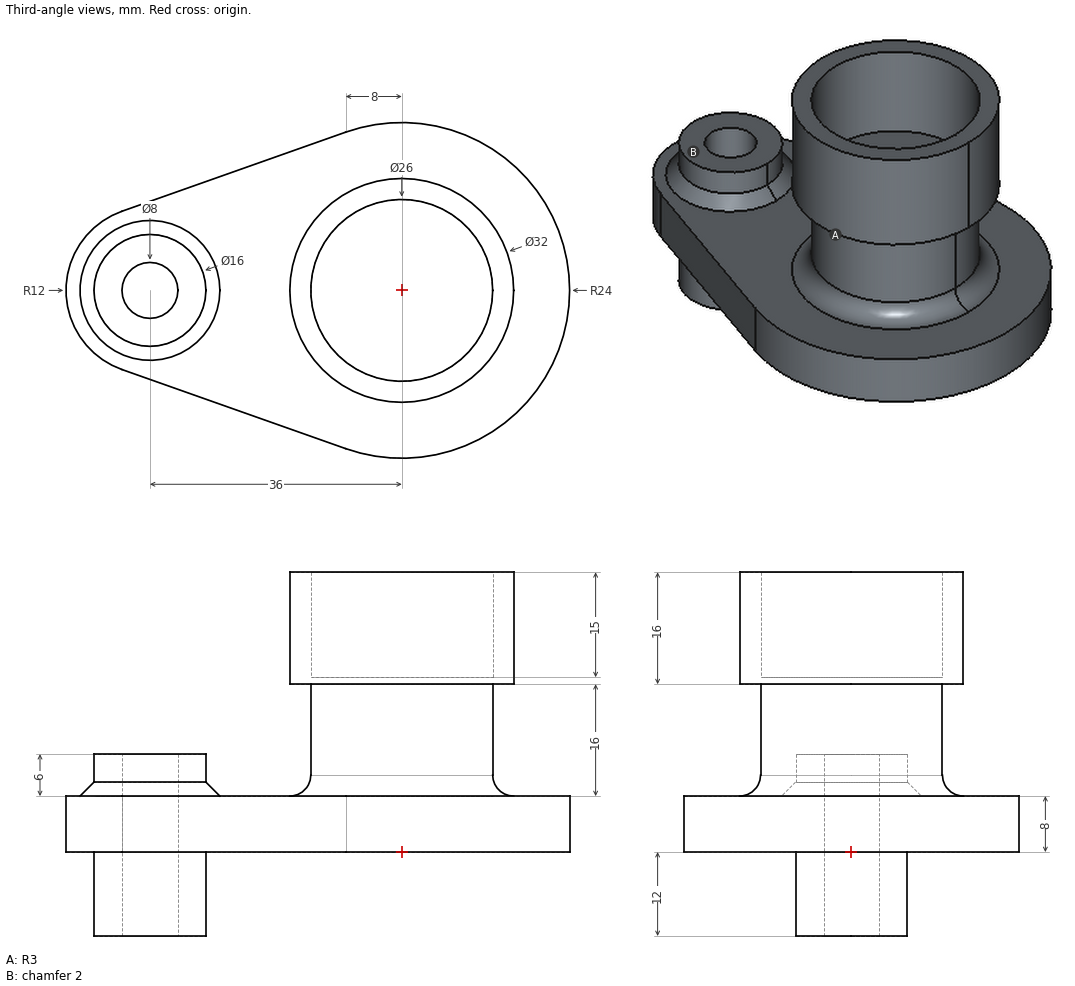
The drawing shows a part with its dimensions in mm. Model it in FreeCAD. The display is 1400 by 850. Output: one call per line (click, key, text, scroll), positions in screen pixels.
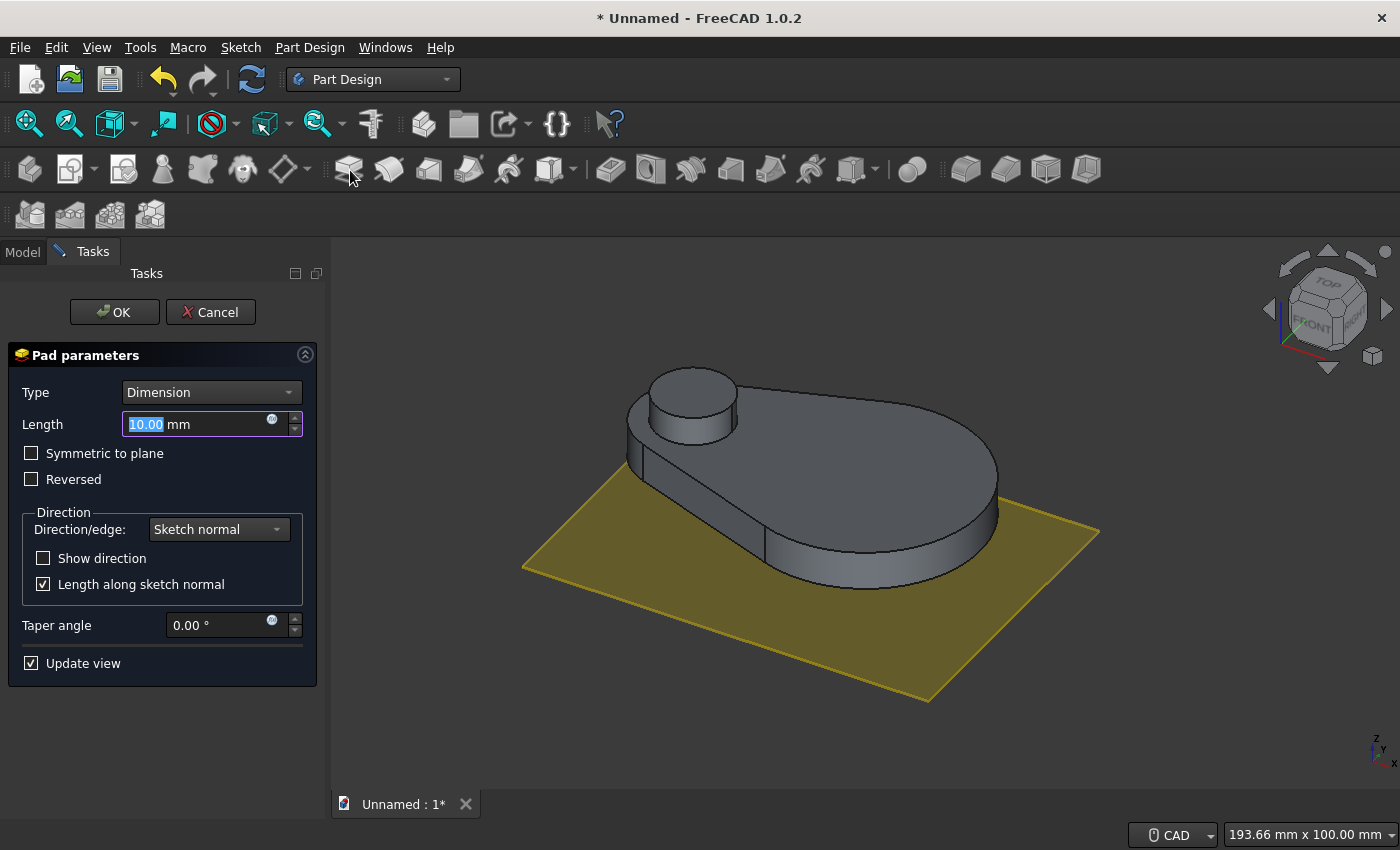
text(12)
key(Tab)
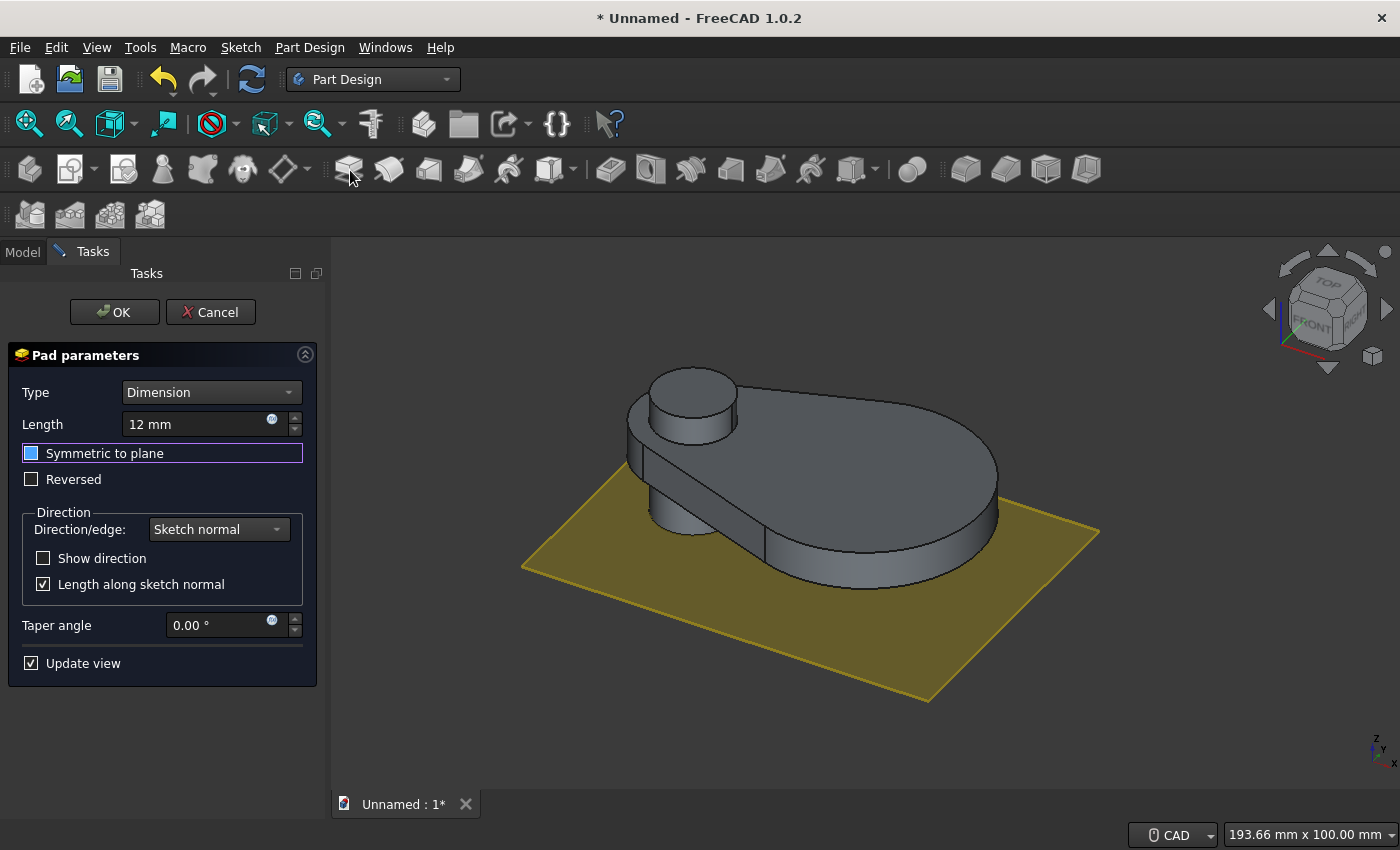
click(115, 312)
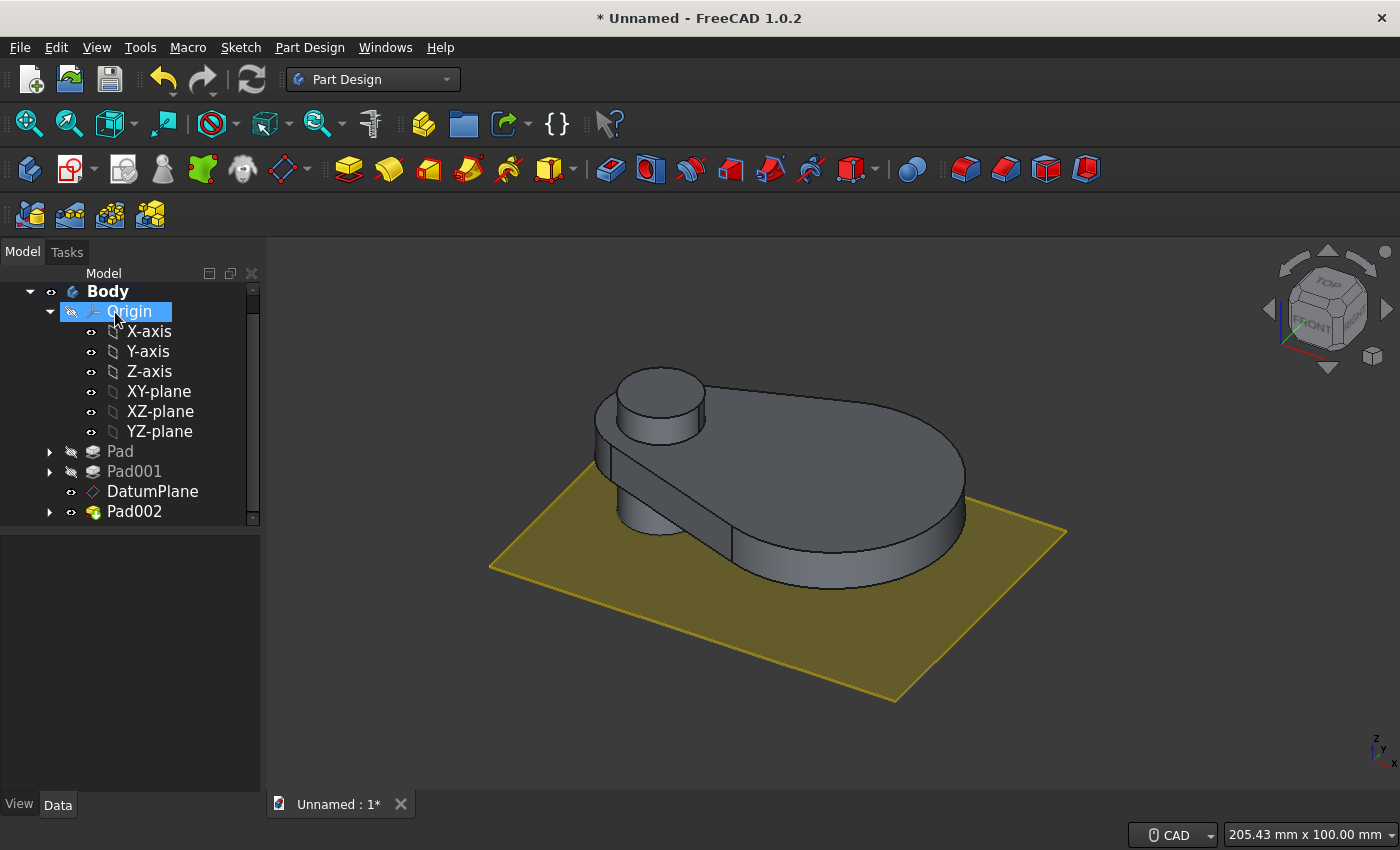
click(116, 492)
key(space)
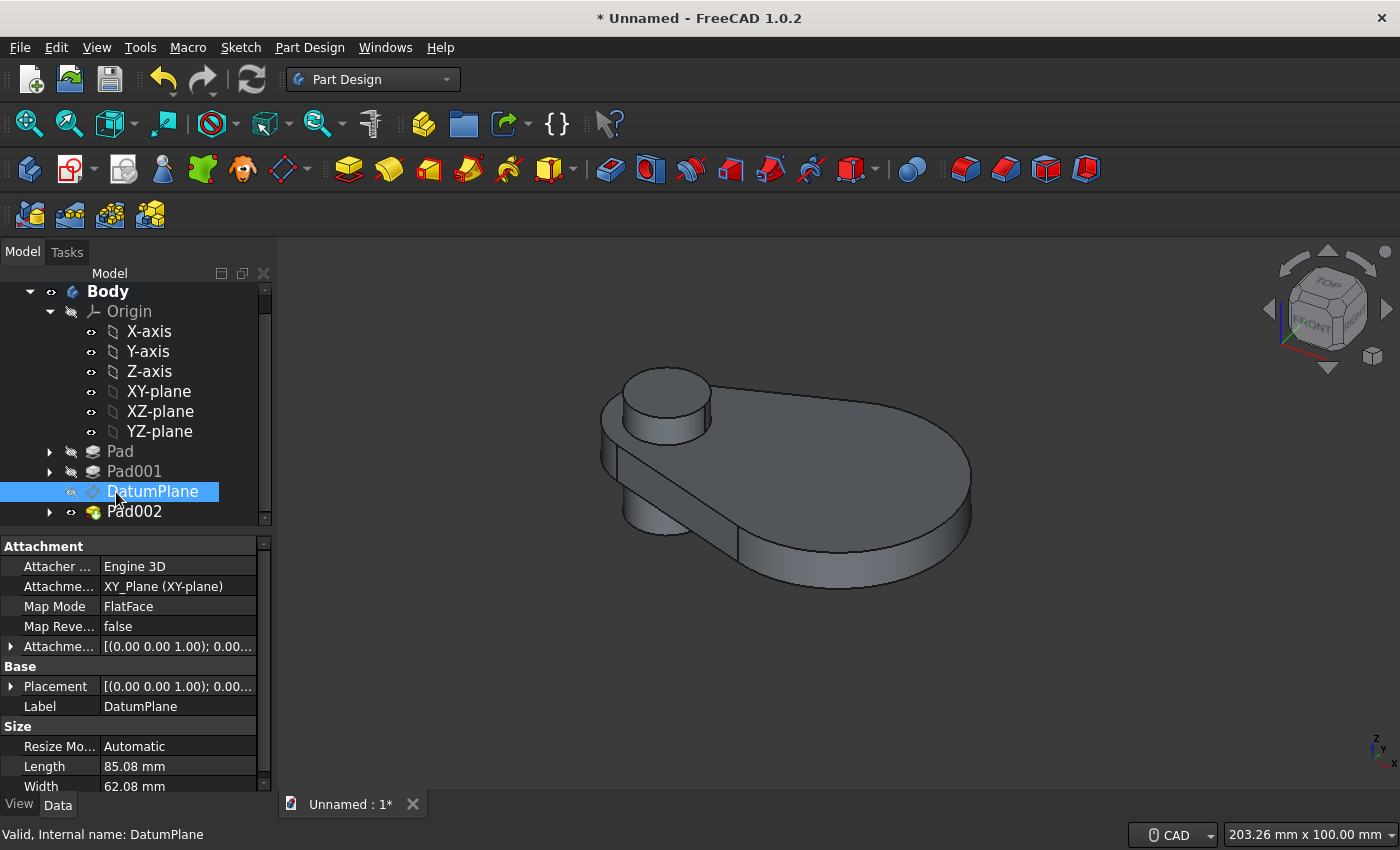
click(831, 473)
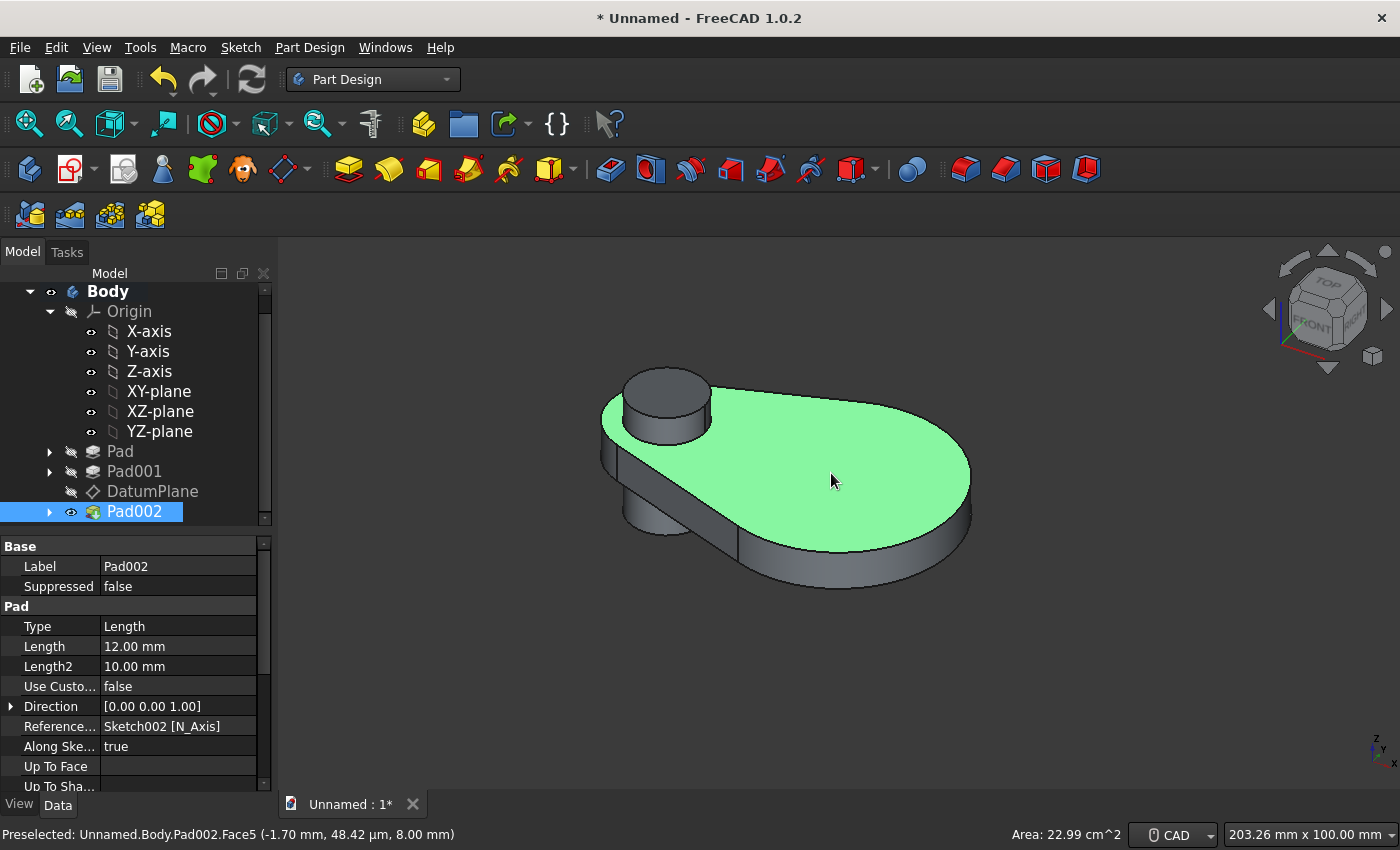
click(70, 170)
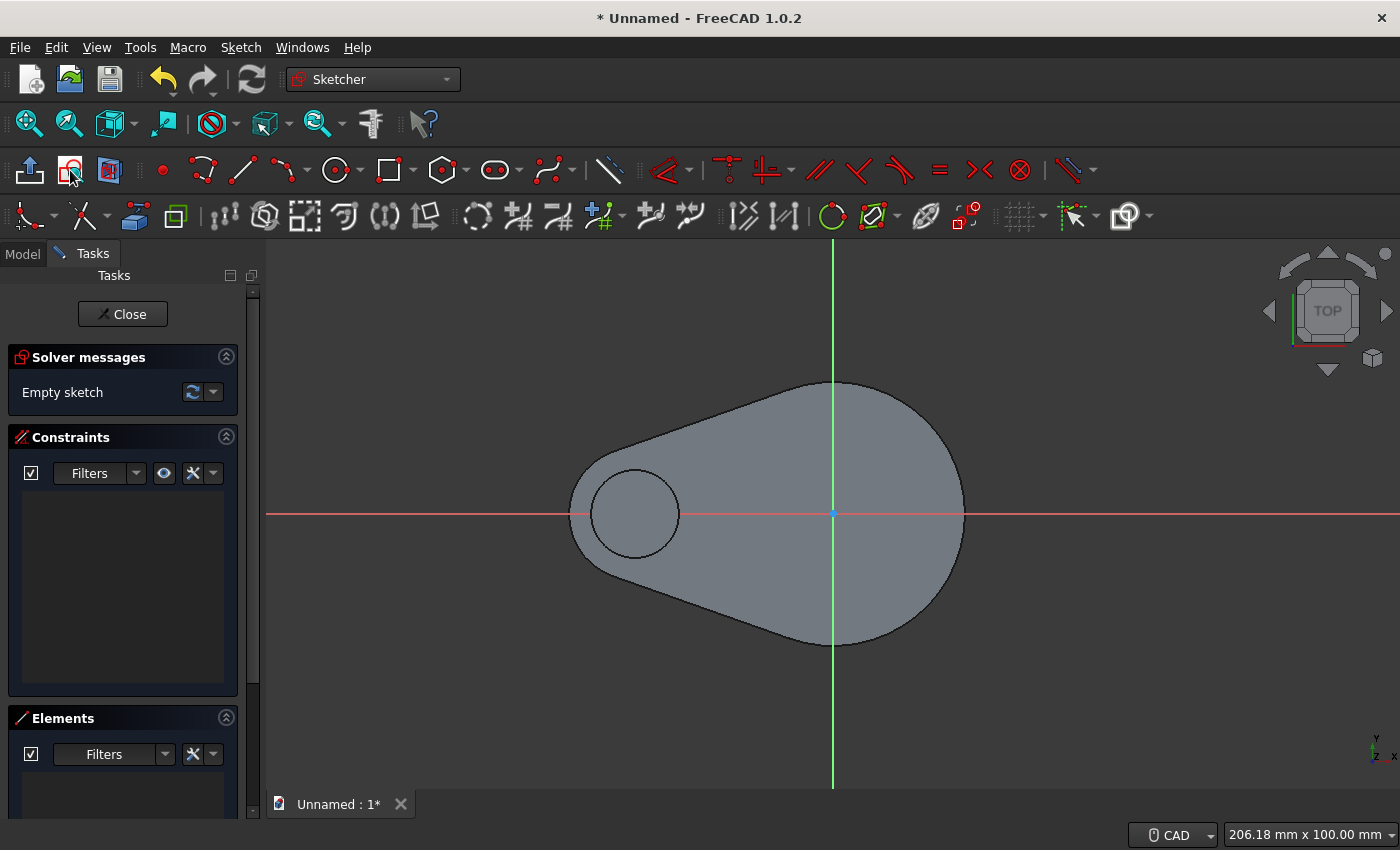
scroll(889, 514, up, 4)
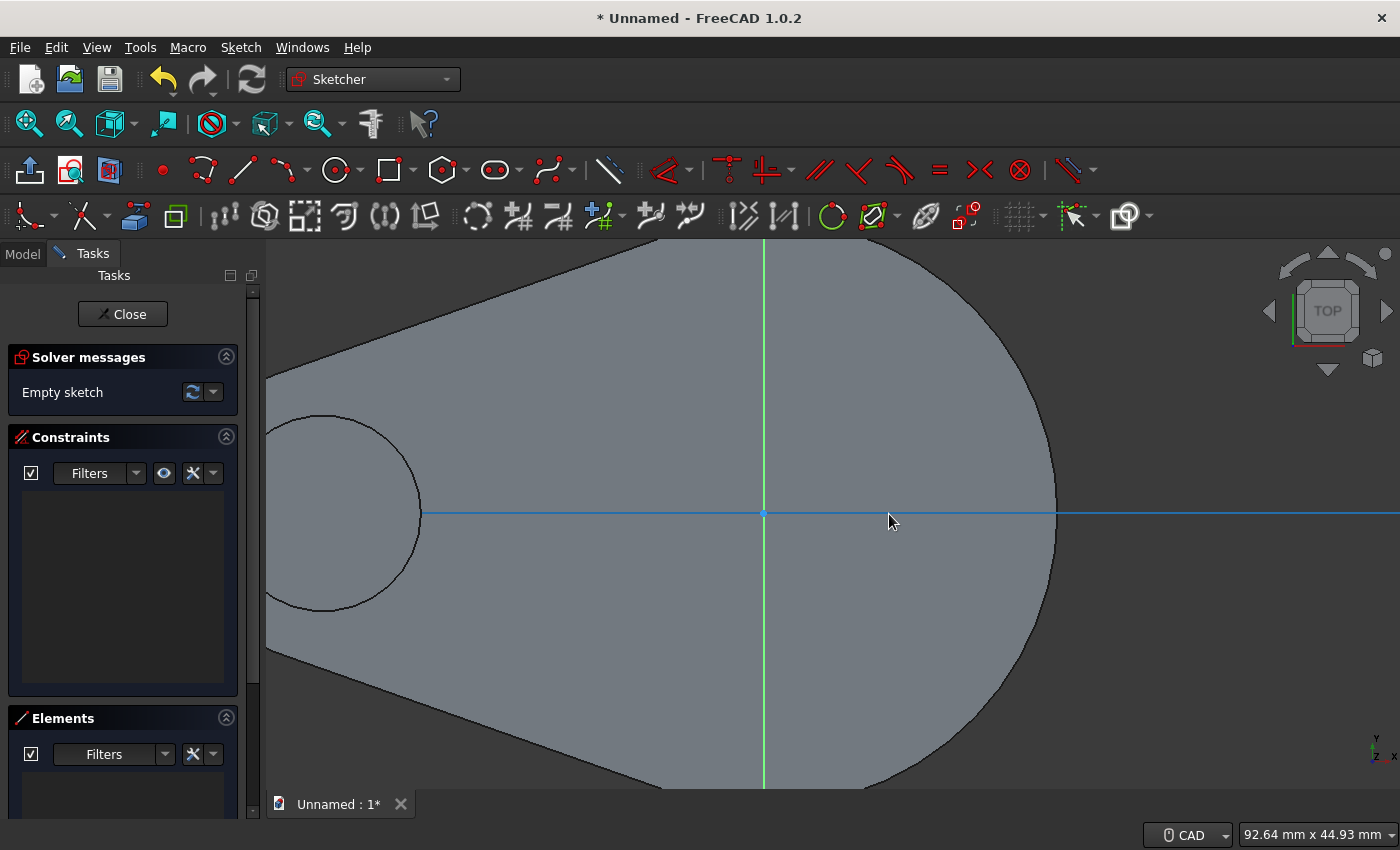
key(g)
key(c)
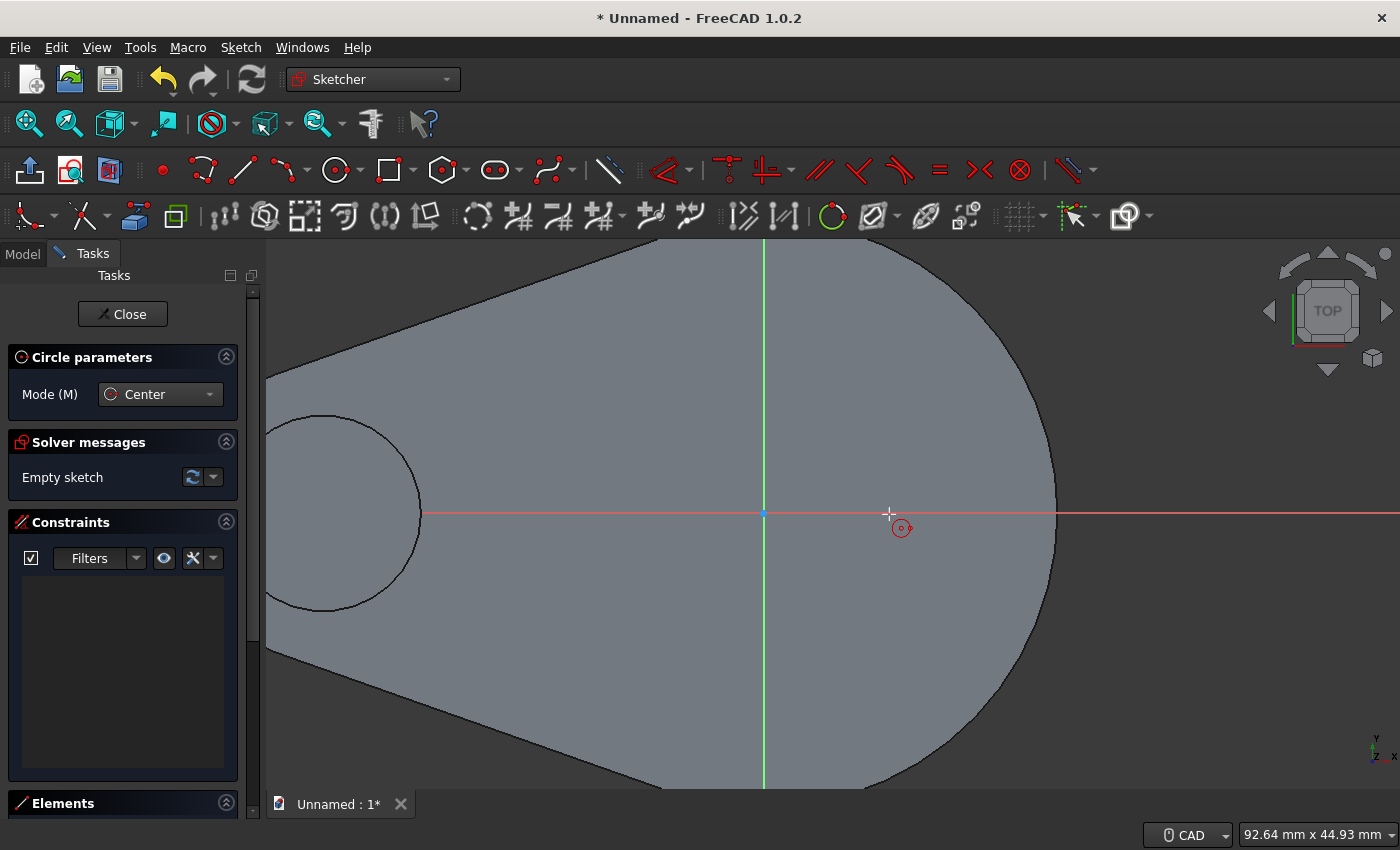
click(764, 513)
move(876, 401)